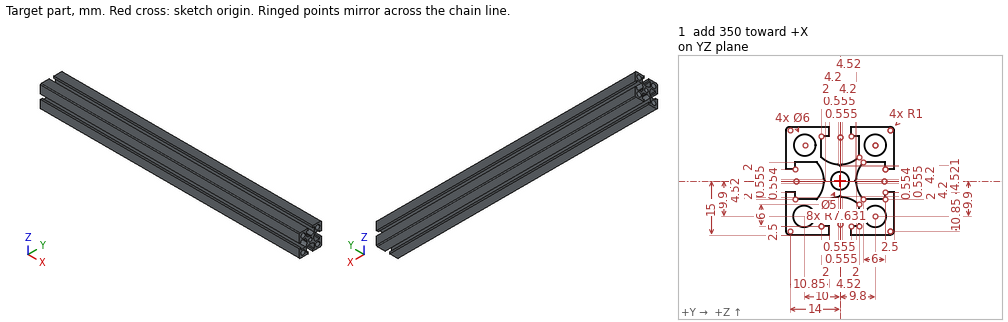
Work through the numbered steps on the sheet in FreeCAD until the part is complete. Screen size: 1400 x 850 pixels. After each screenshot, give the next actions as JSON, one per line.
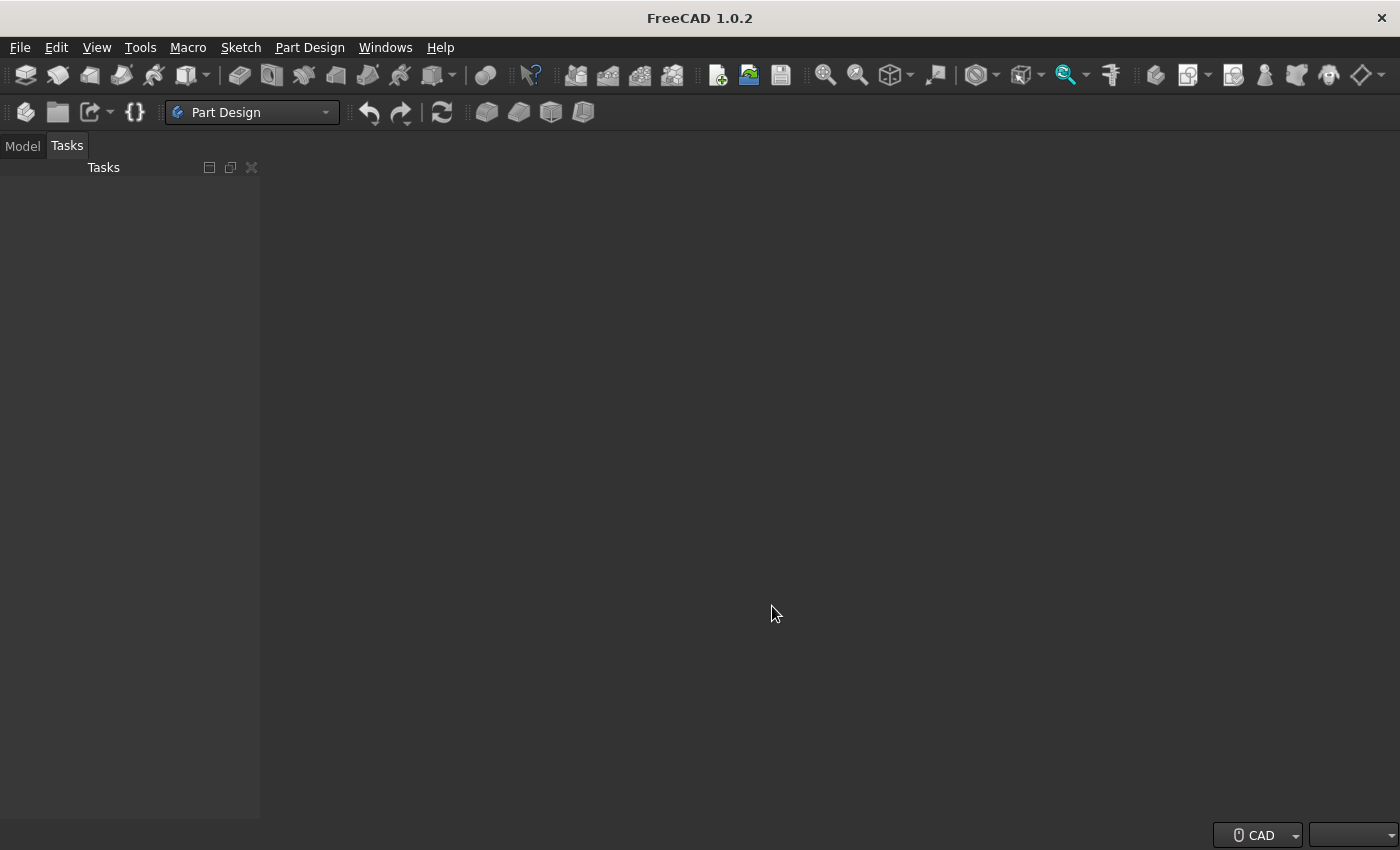
{"action": "left_click", "coordinate": [718, 76]}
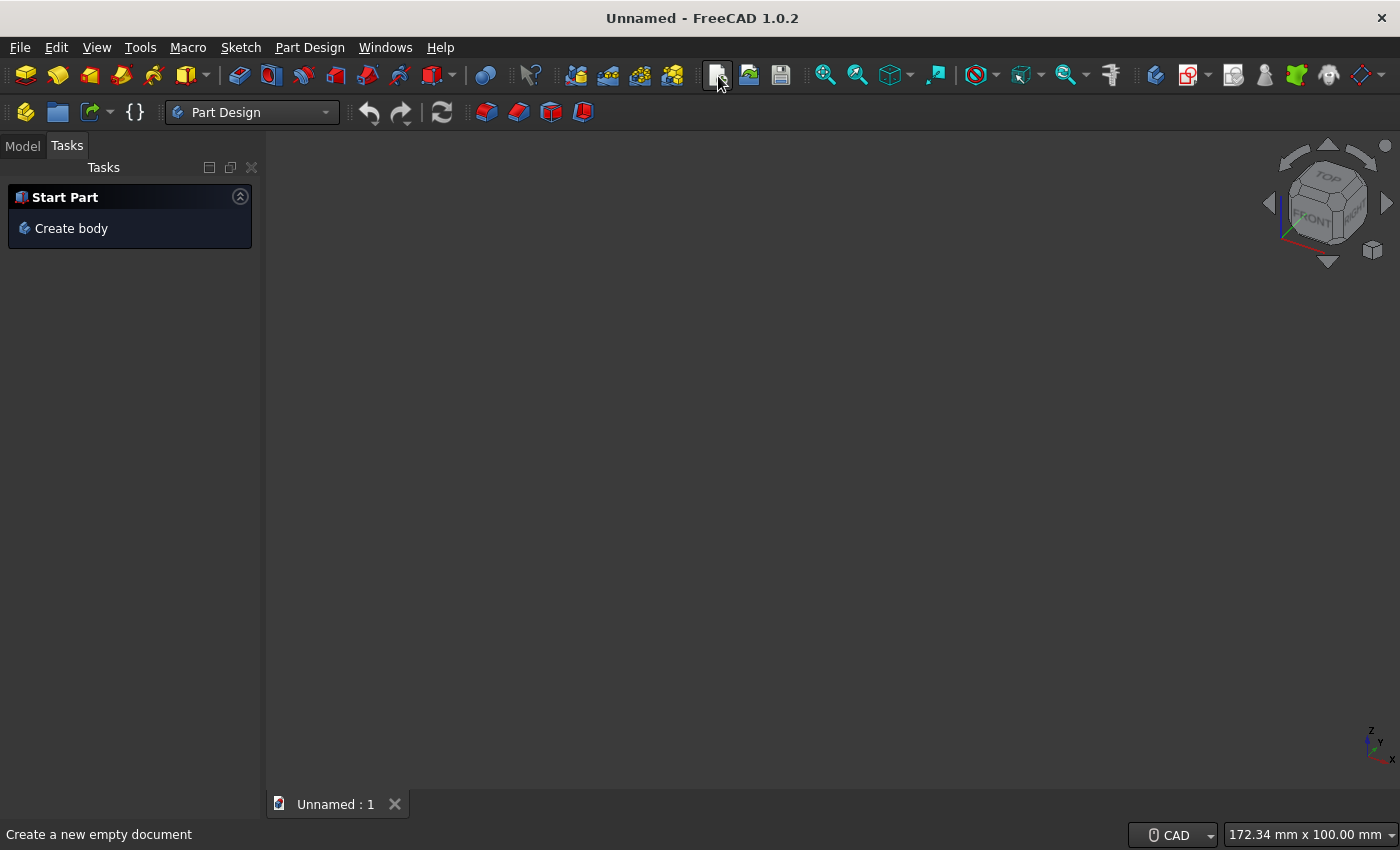
{"action": "left_click", "coordinate": [1188, 76]}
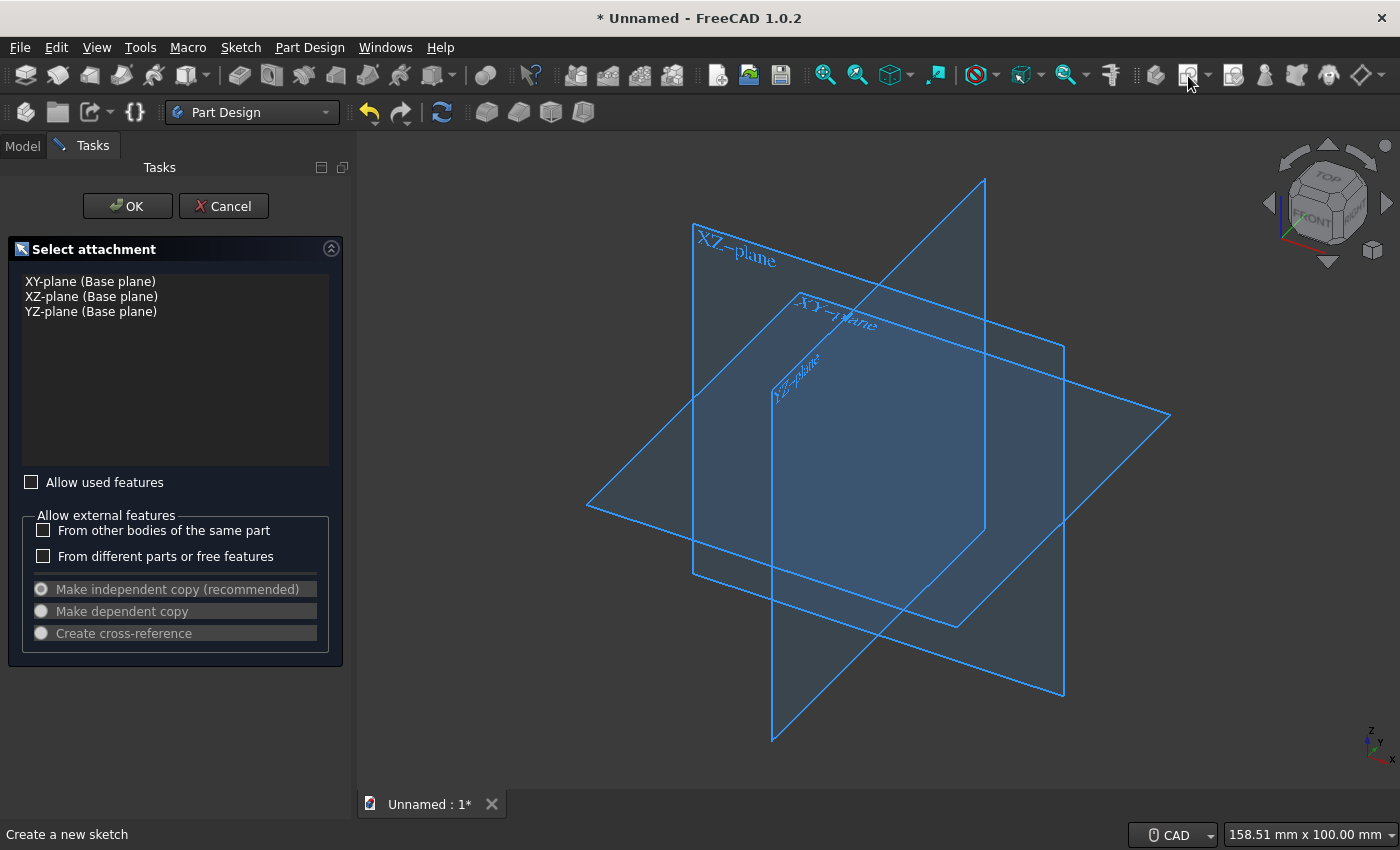
{"action": "left_click", "coordinate": [82, 312]}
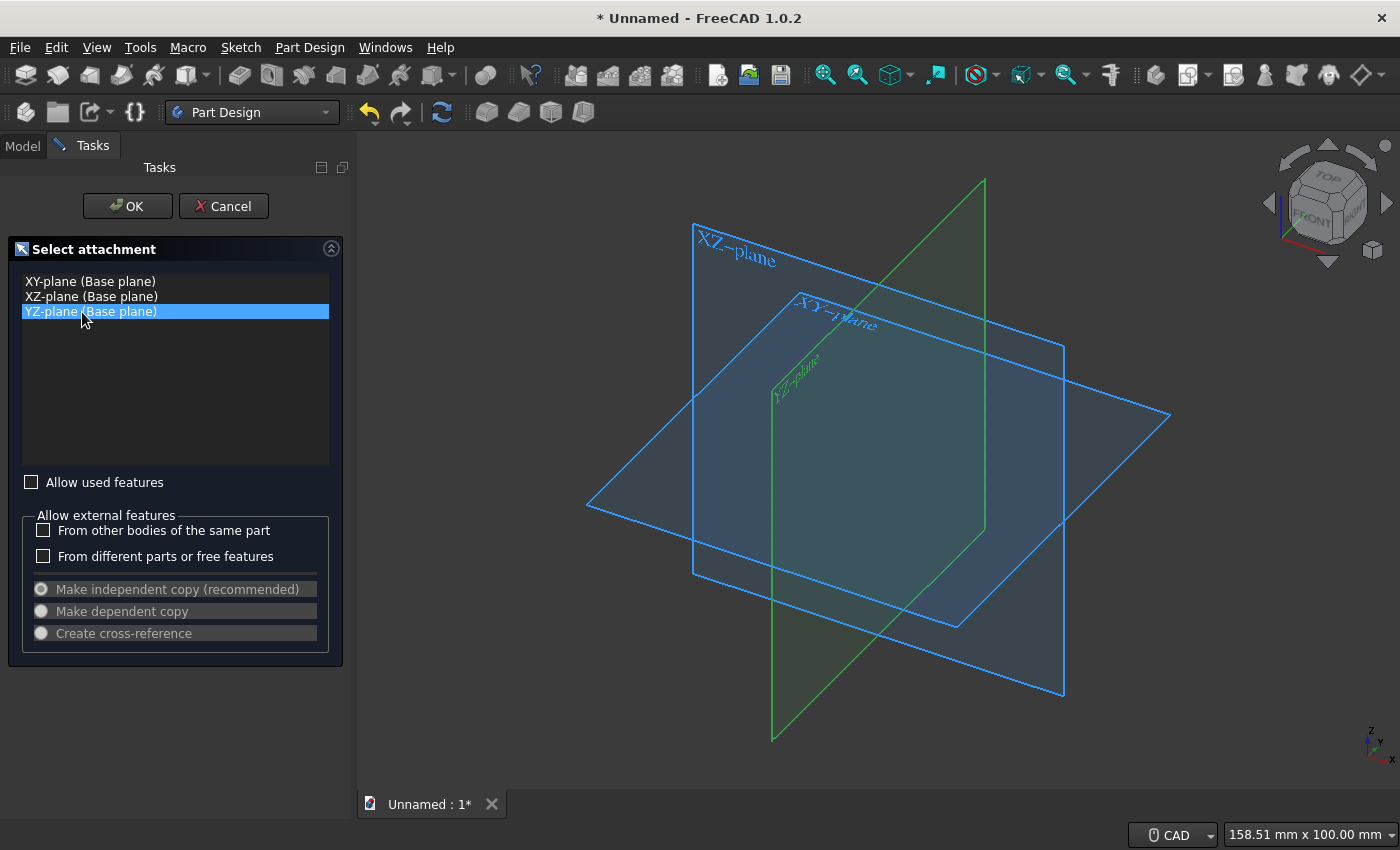
{"action": "left_click", "coordinate": [128, 206]}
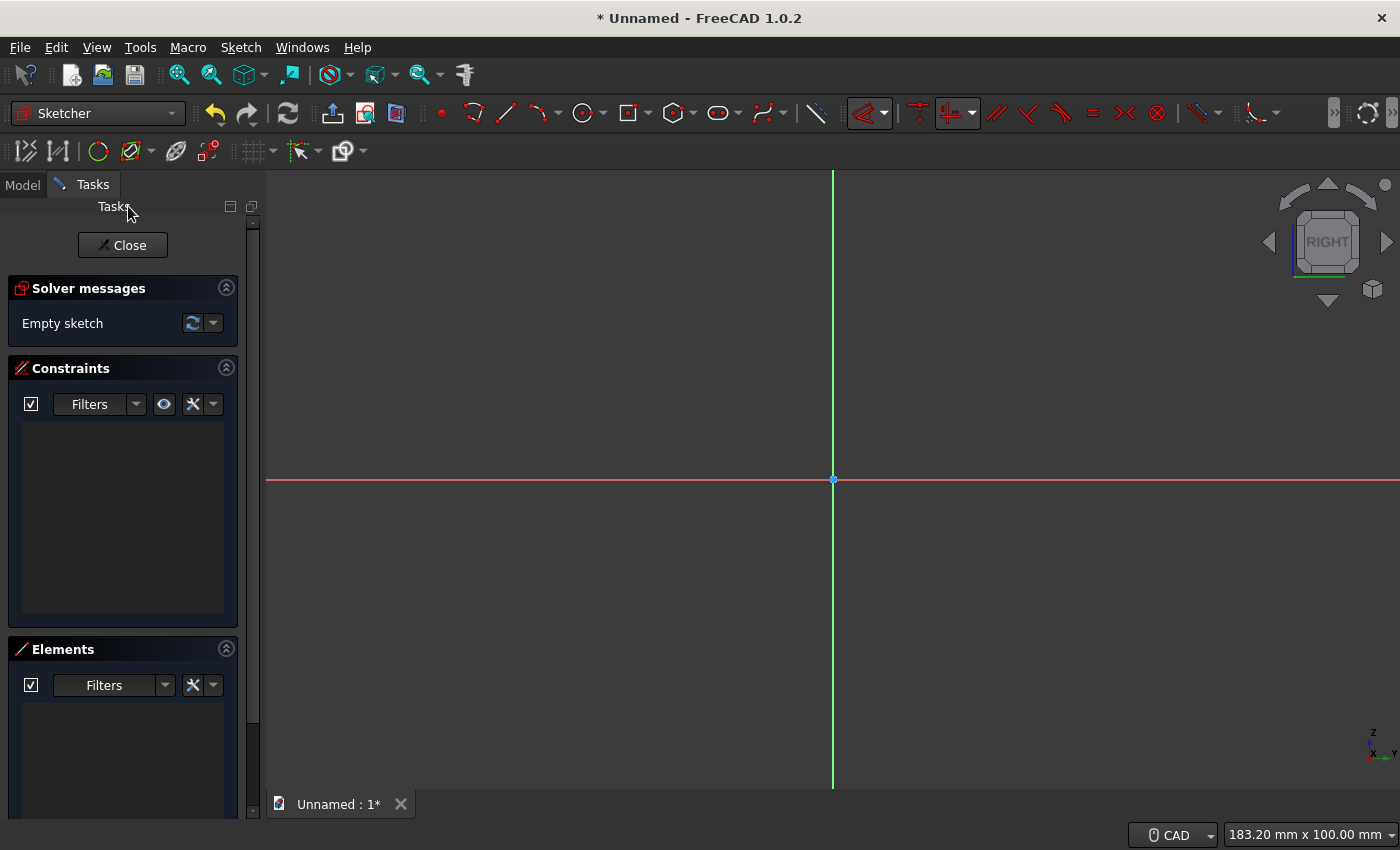
{"action": "scroll", "coordinate": [889, 480], "scroll_direction": "up", "scroll_amount": 4}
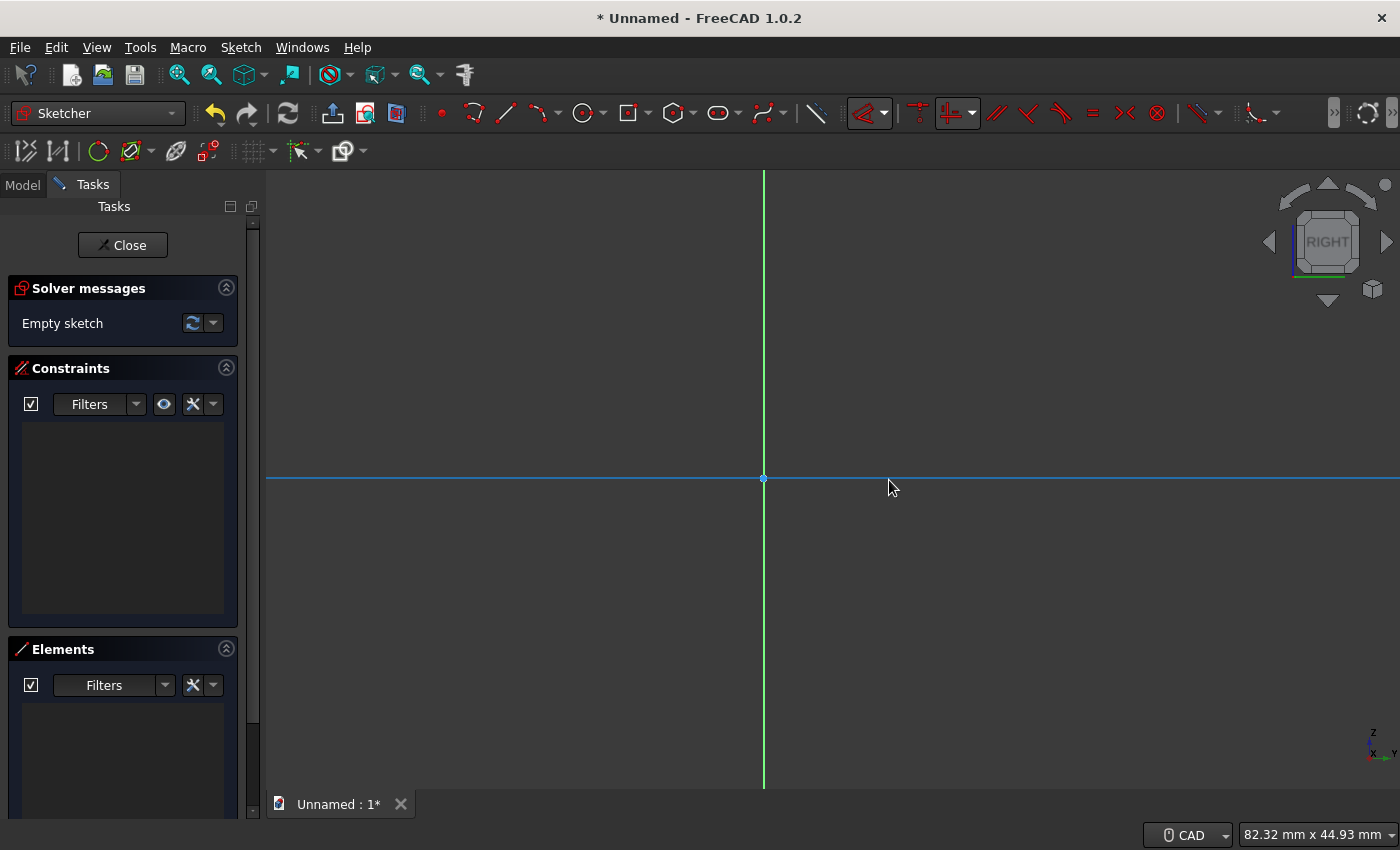
{"action": "left_click", "coordinate": [474, 114]}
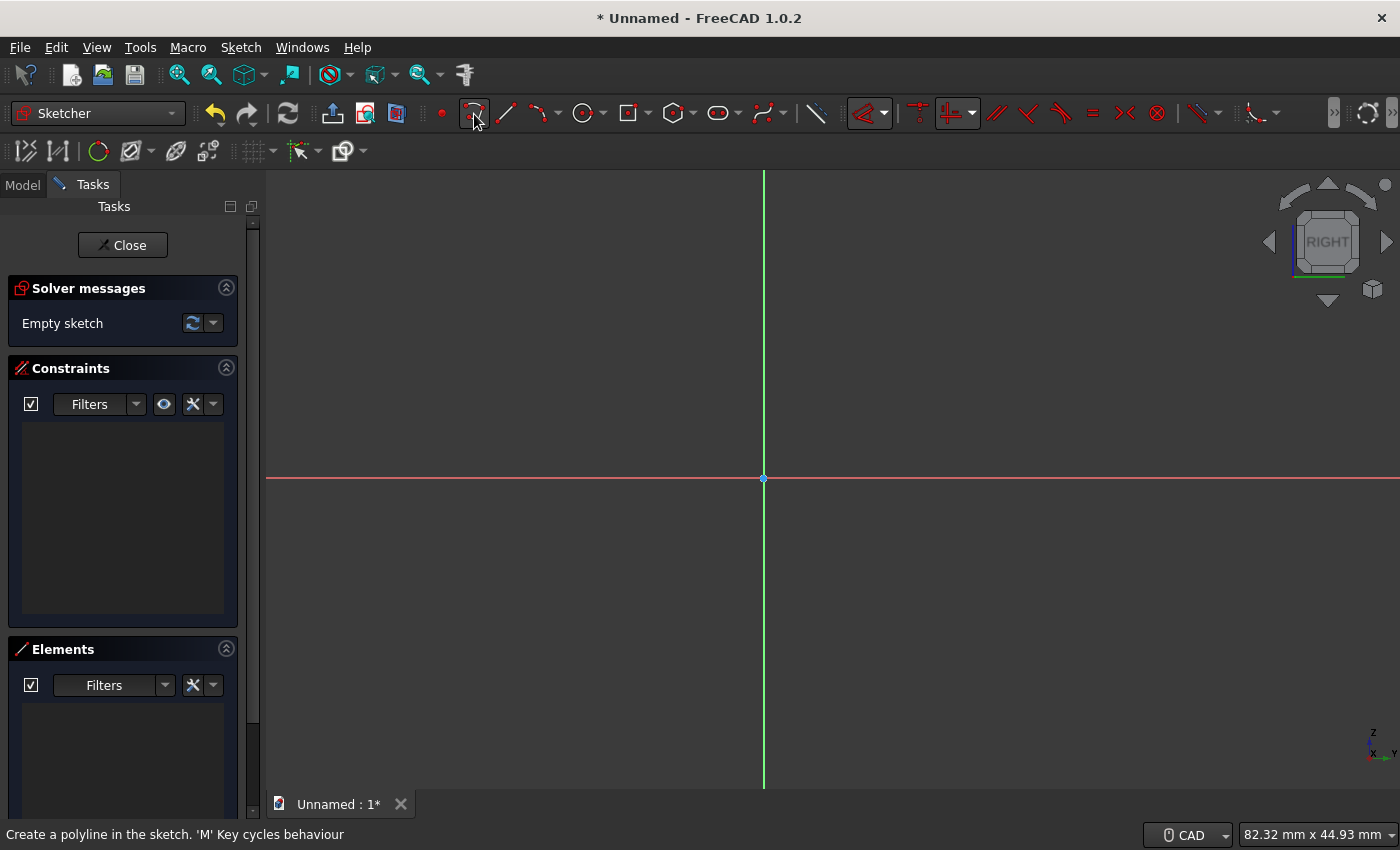
{"action": "left_click", "coordinate": [571, 685]}
{"action": "left_click", "coordinate": [720, 685]}
{"action": "left_click", "coordinate": [720, 650]}
{"action": "left_click", "coordinate": [693, 650]}
{"action": "left_click", "coordinate": [693, 568]}
{"action": "right_click", "coordinate": [693, 568]}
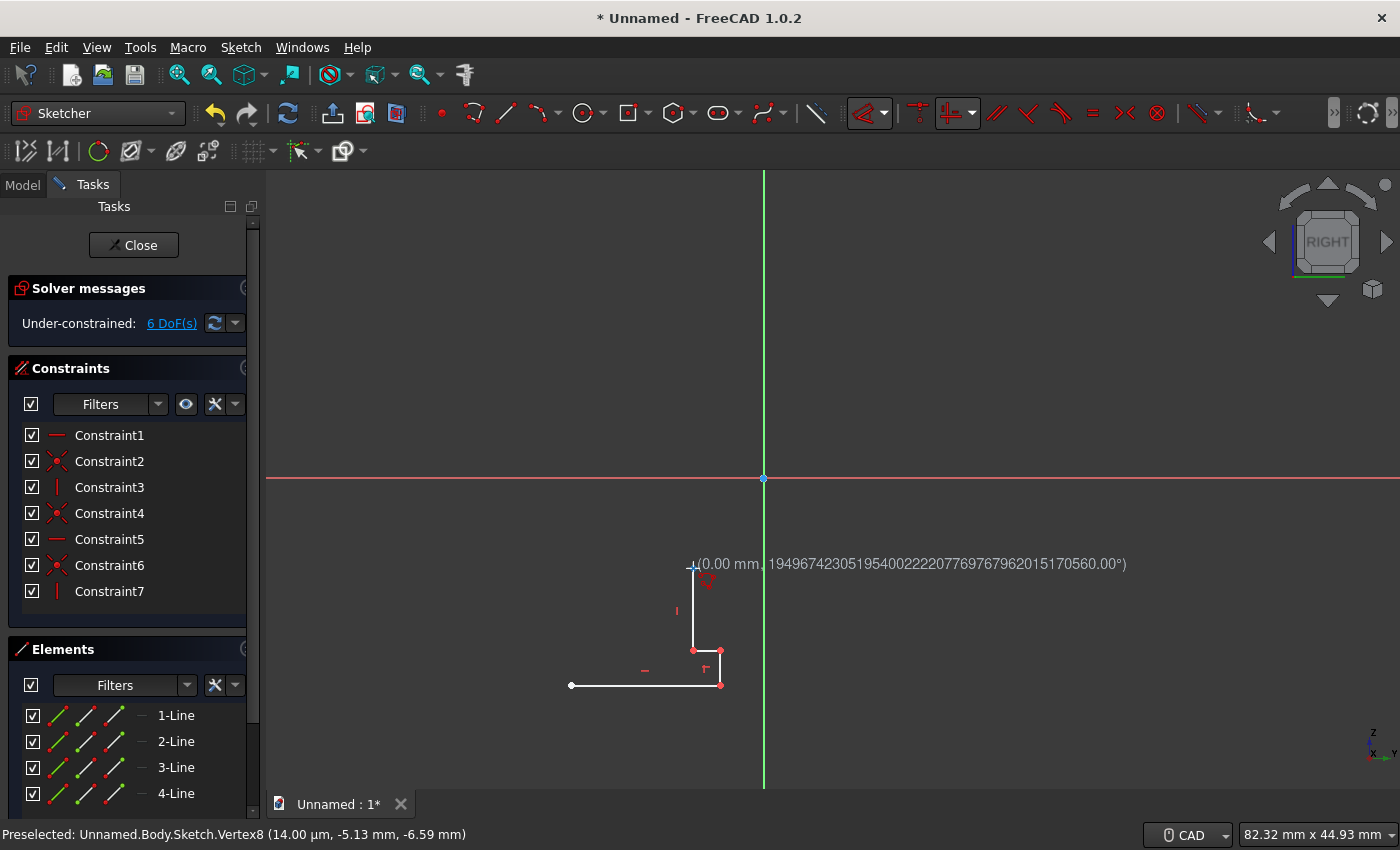
{"action": "scroll", "coordinate": [756, 541], "scroll_direction": "up", "scroll_amount": 4}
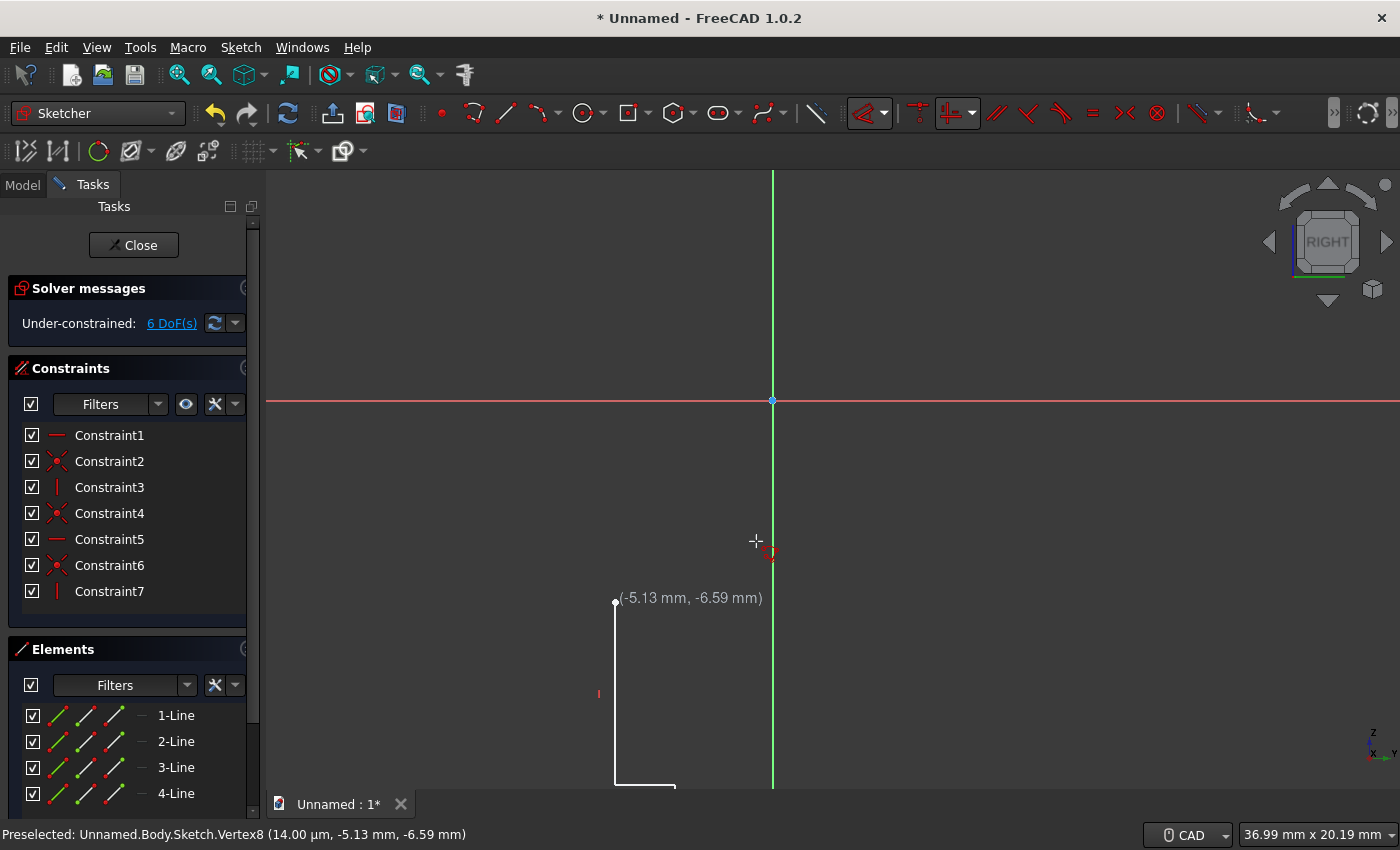
{"action": "left_click", "coordinate": [756, 539]}
{"action": "left_click", "coordinate": [773, 529]}
{"action": "left_click", "coordinate": [790, 539]}
{"action": "right_click", "coordinate": [790, 539]}